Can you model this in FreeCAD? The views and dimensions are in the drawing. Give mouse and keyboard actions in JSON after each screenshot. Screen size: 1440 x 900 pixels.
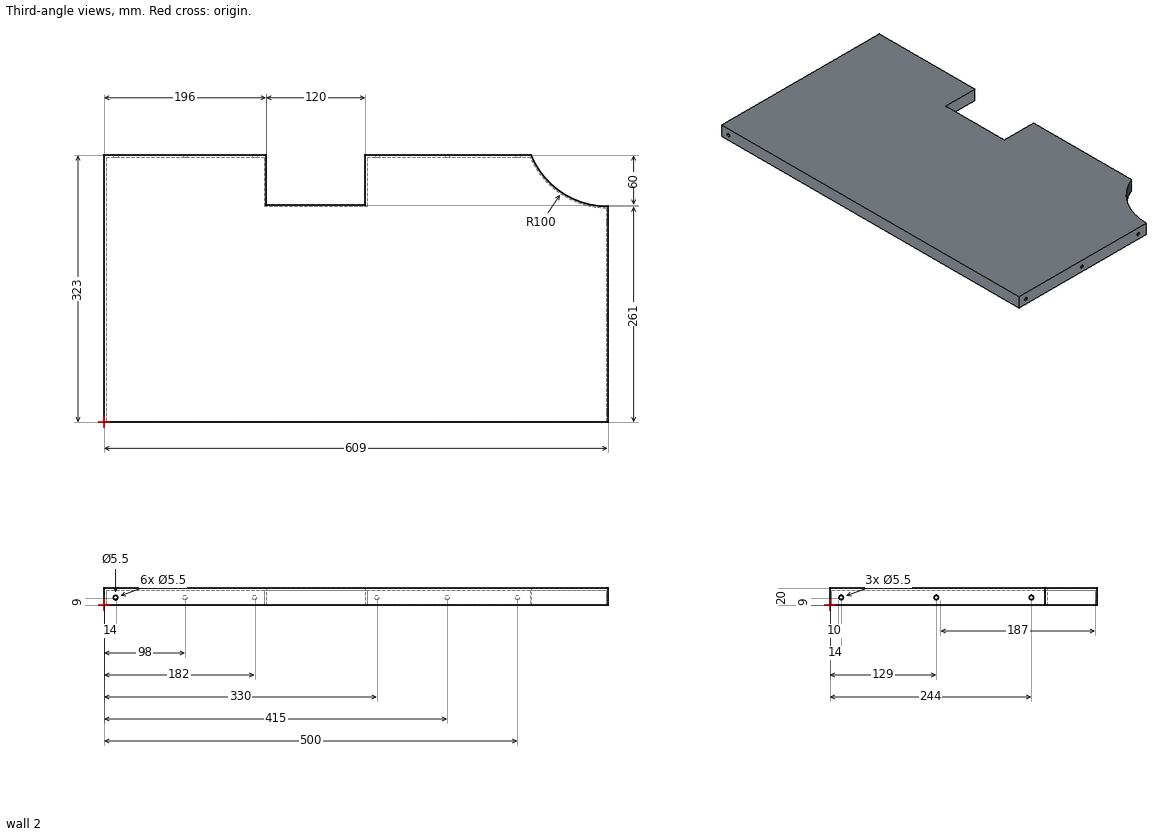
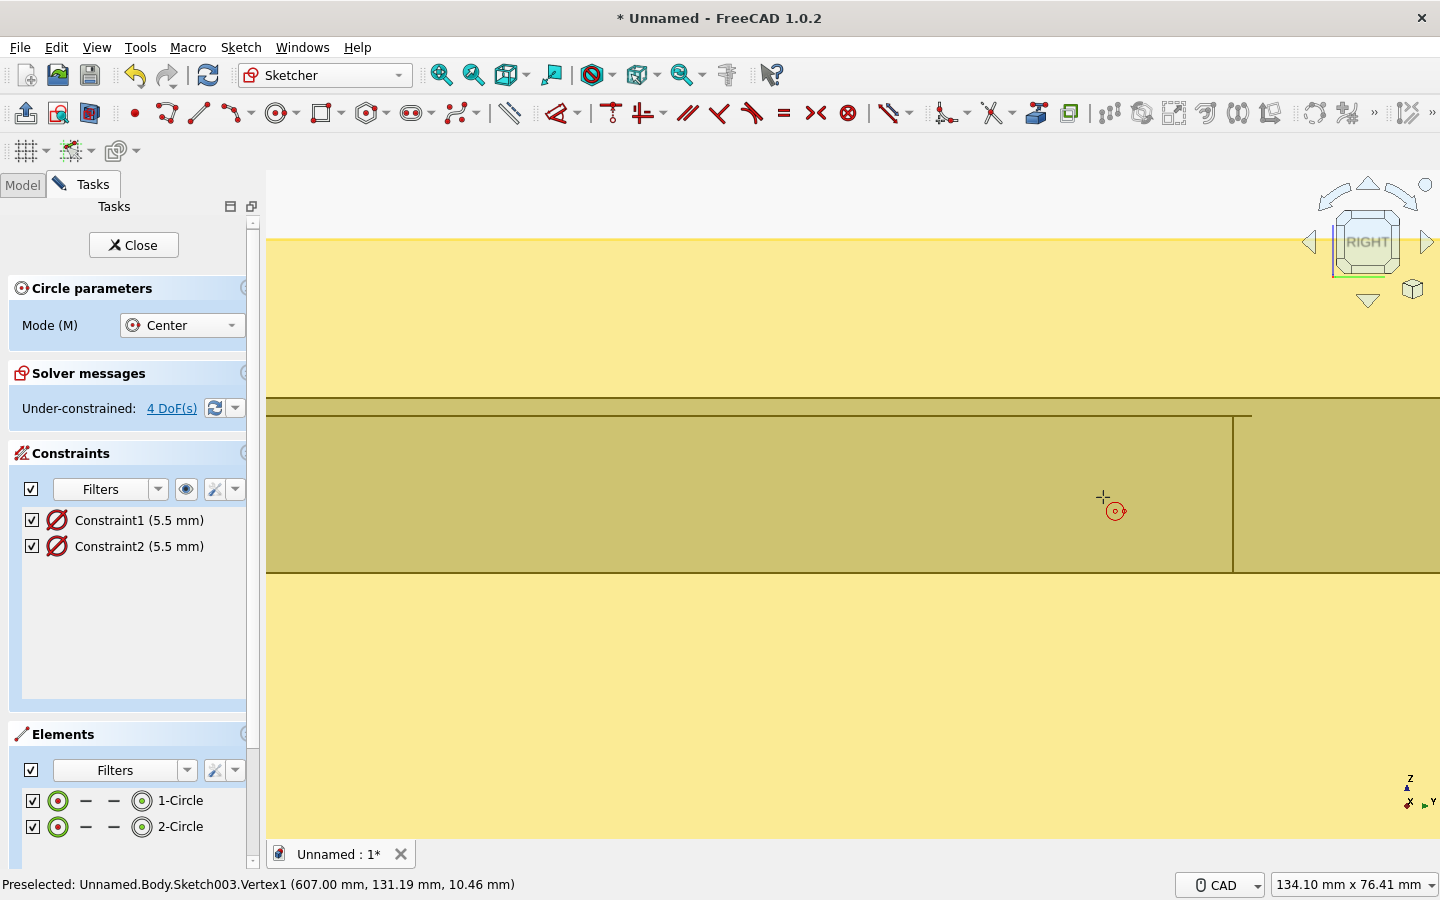
{"action": "left_click", "coordinate": [1102, 495]}
{"action": "mouse_move", "coordinate": [1119, 478]}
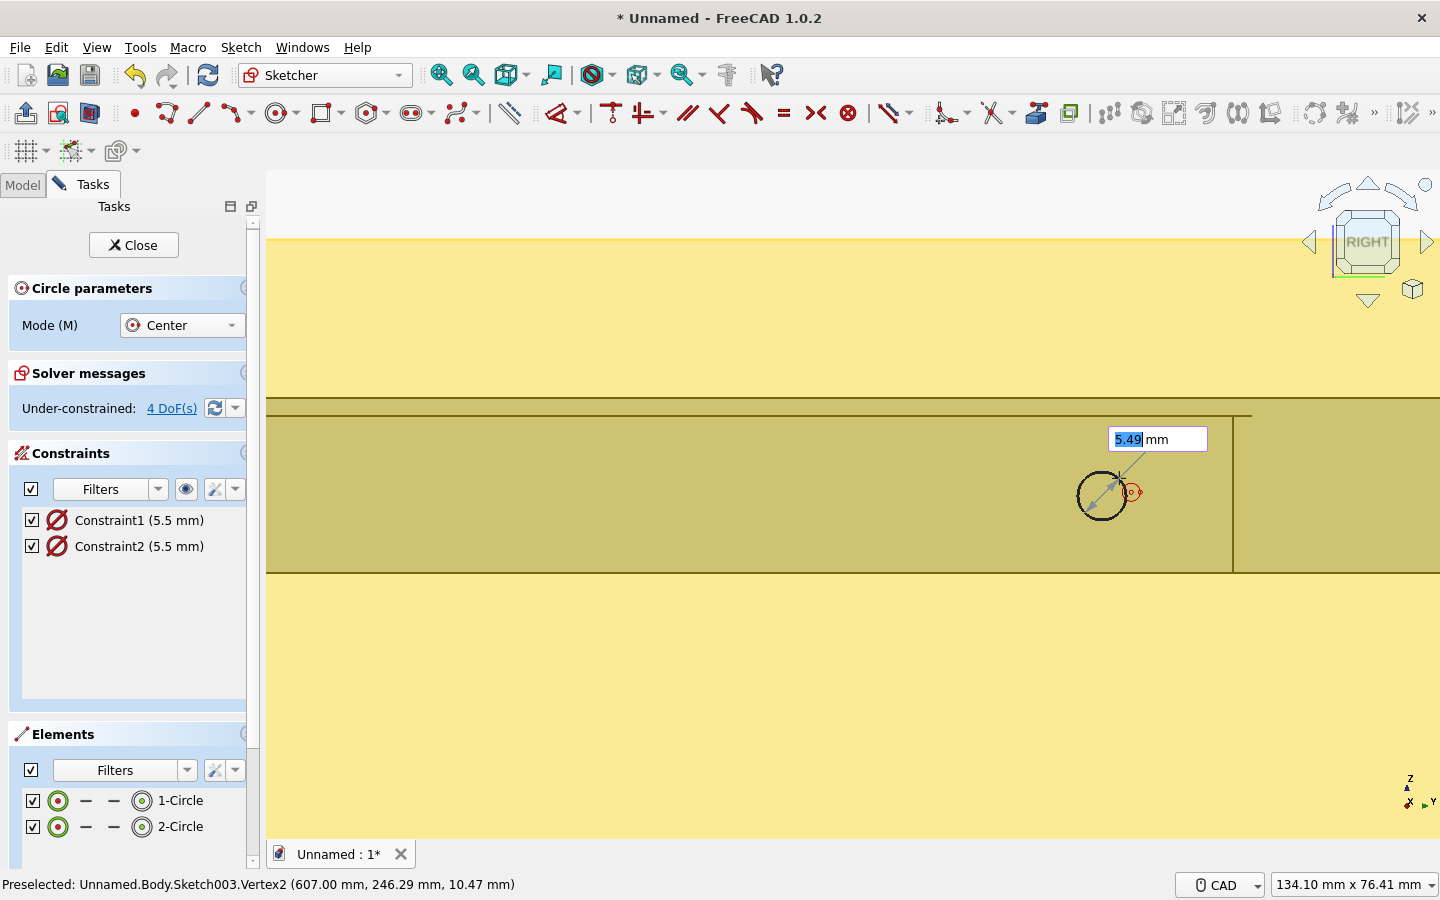
{"action": "type", "text": "5.5"}
{"action": "key", "text": "Return"}
{"action": "key", "text": "Escape"}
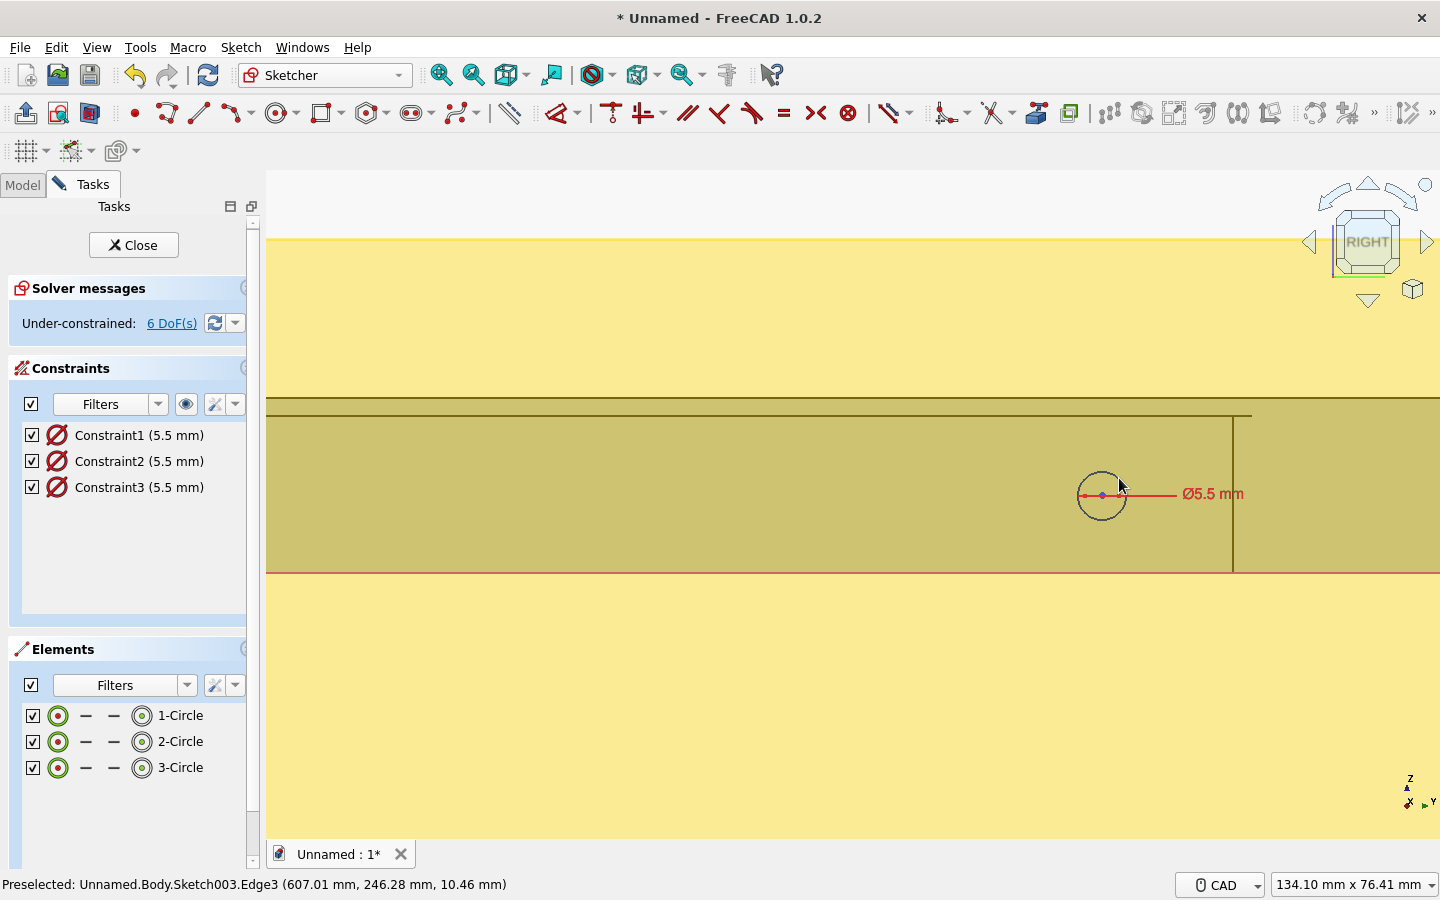
{"action": "key", "text": "d"}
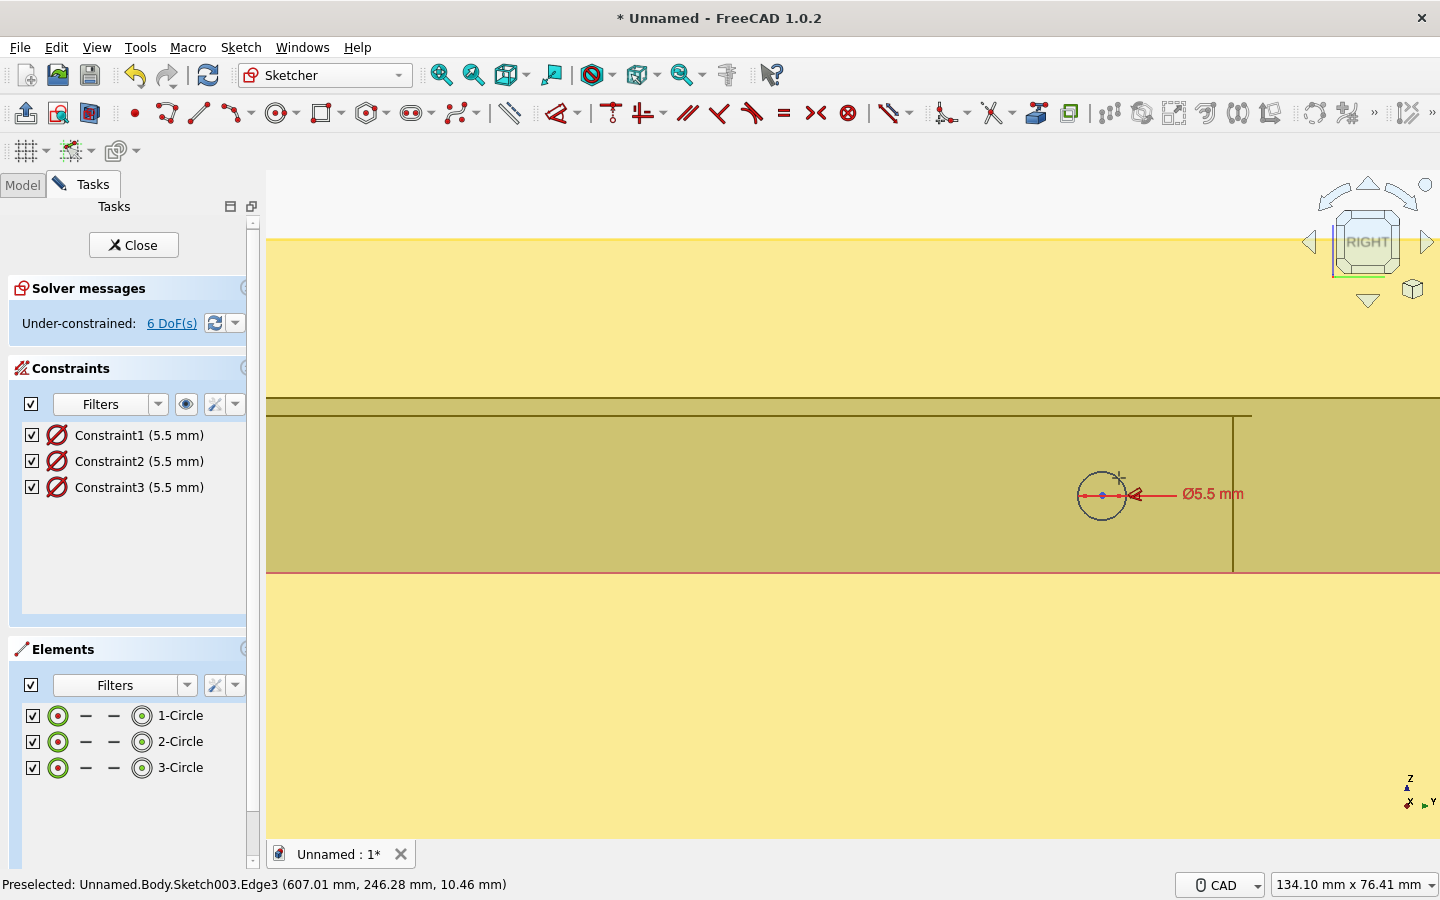
{"action": "scroll", "coordinate": [1103, 497], "scroll_direction": "down", "scroll_amount": 6}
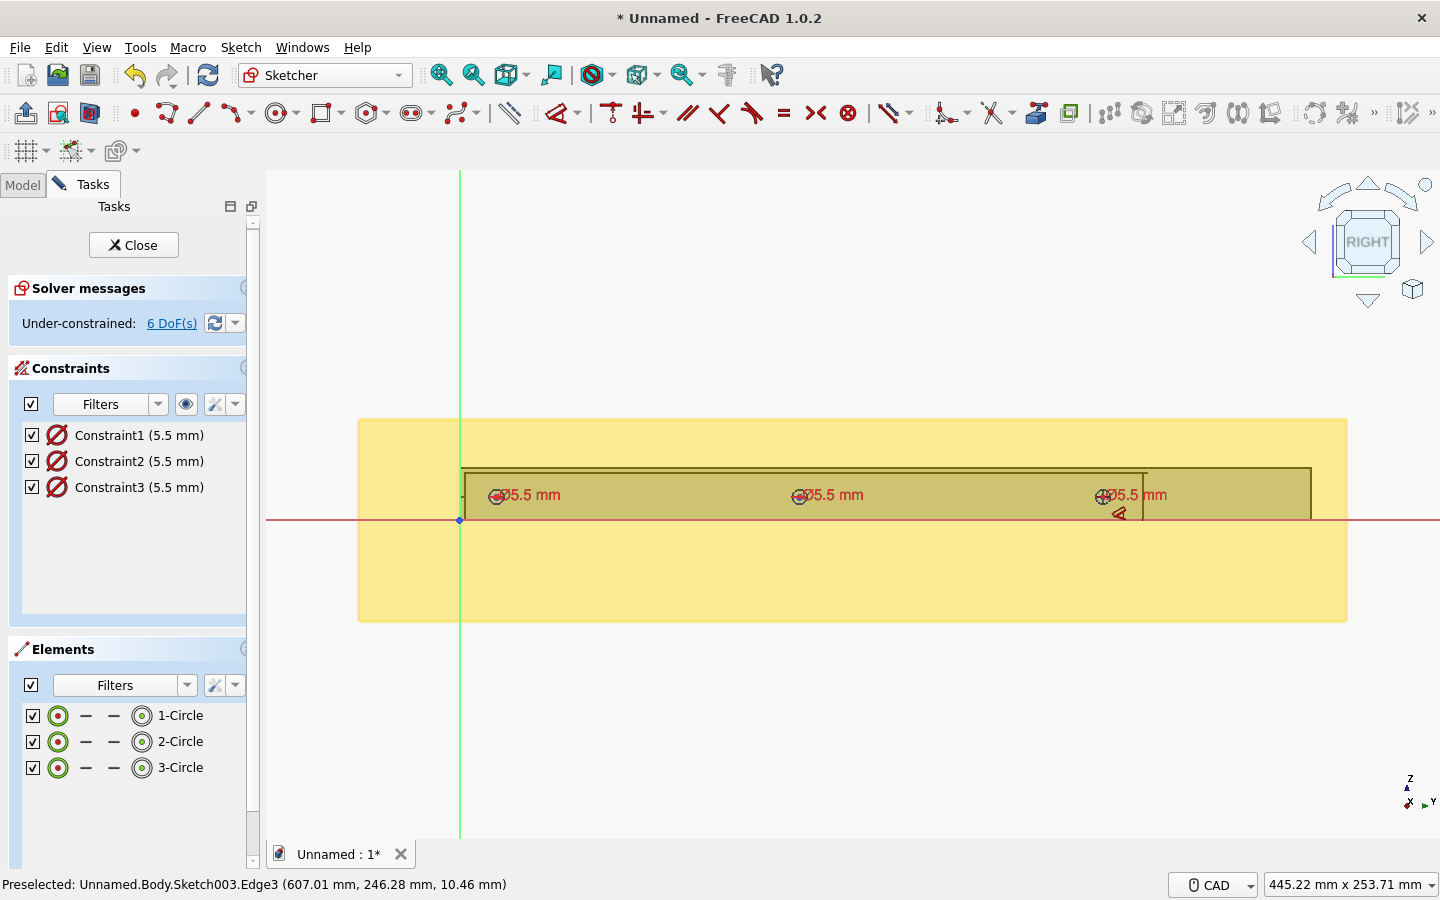
{"action": "scroll", "coordinate": [497, 497], "scroll_direction": "up", "scroll_amount": 3}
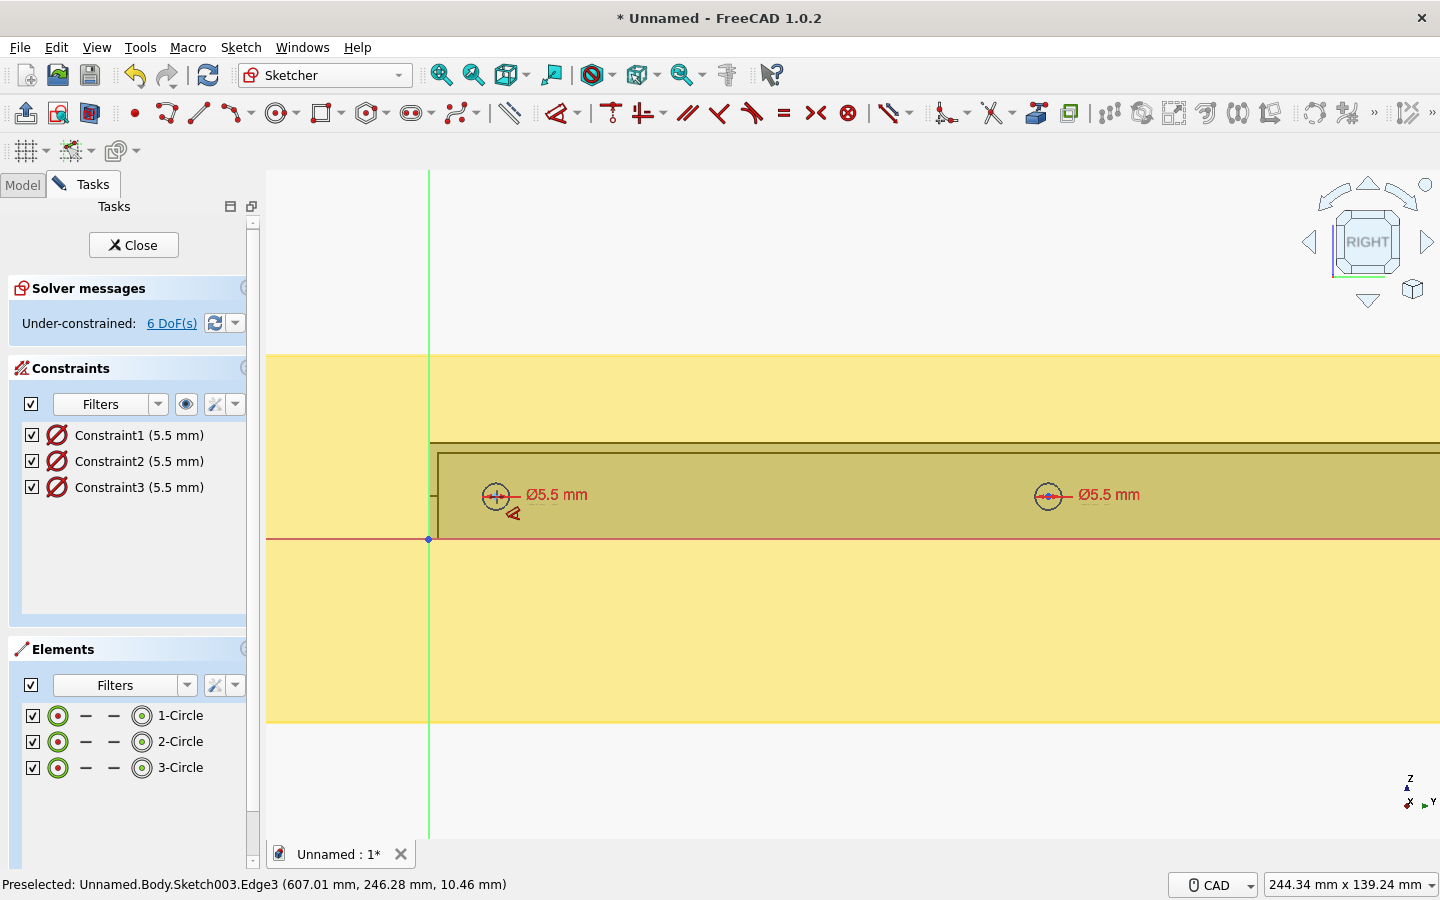
{"action": "left_click", "coordinate": [496, 497]}
{"action": "left_click", "coordinate": [395, 518]}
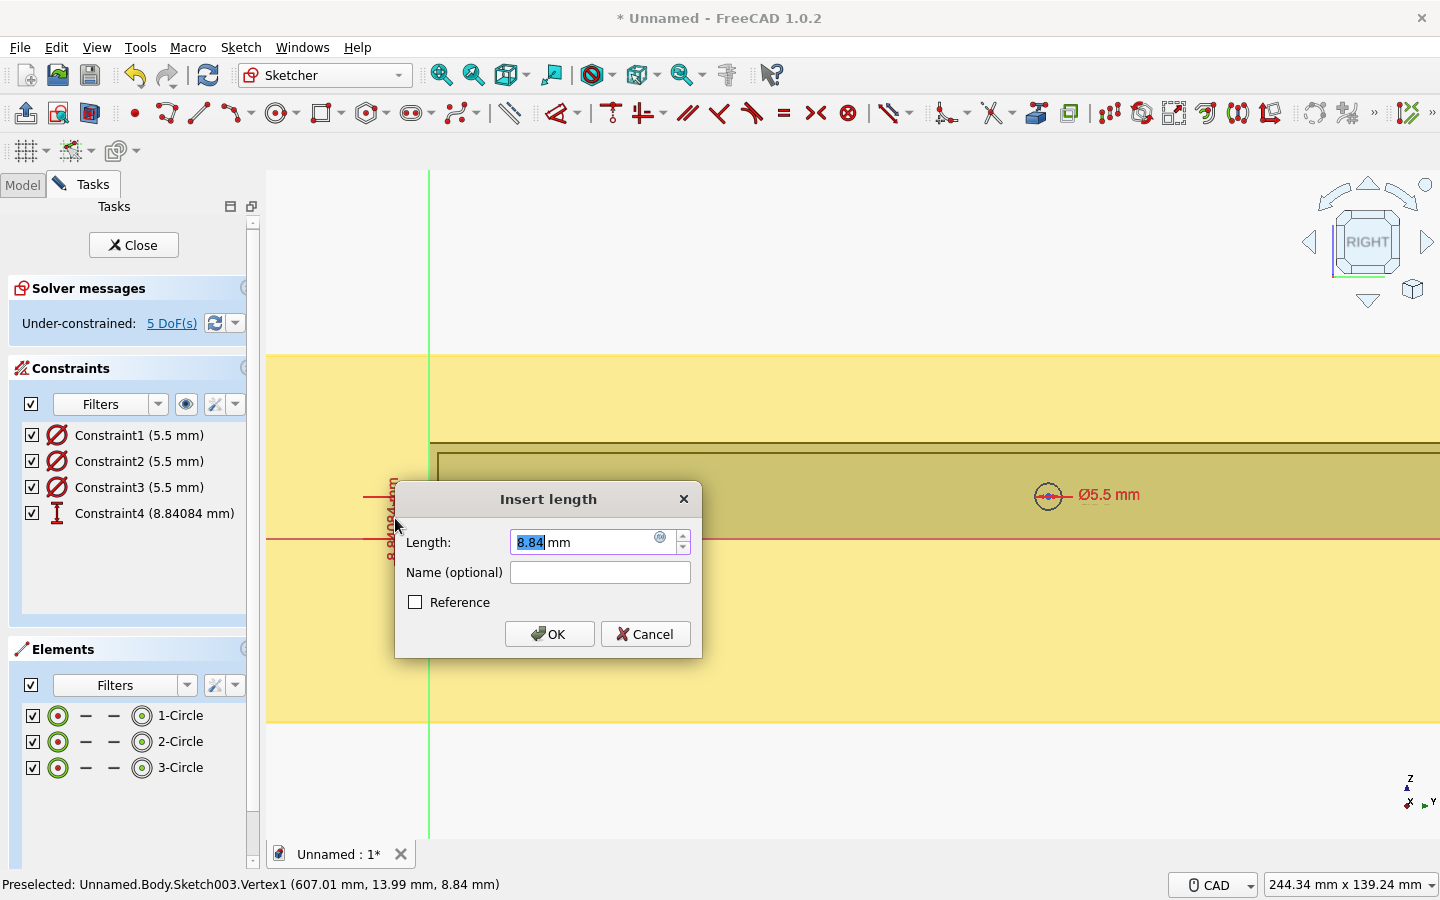
{"action": "type", "text": "9"}
{"action": "key", "text": "Return"}